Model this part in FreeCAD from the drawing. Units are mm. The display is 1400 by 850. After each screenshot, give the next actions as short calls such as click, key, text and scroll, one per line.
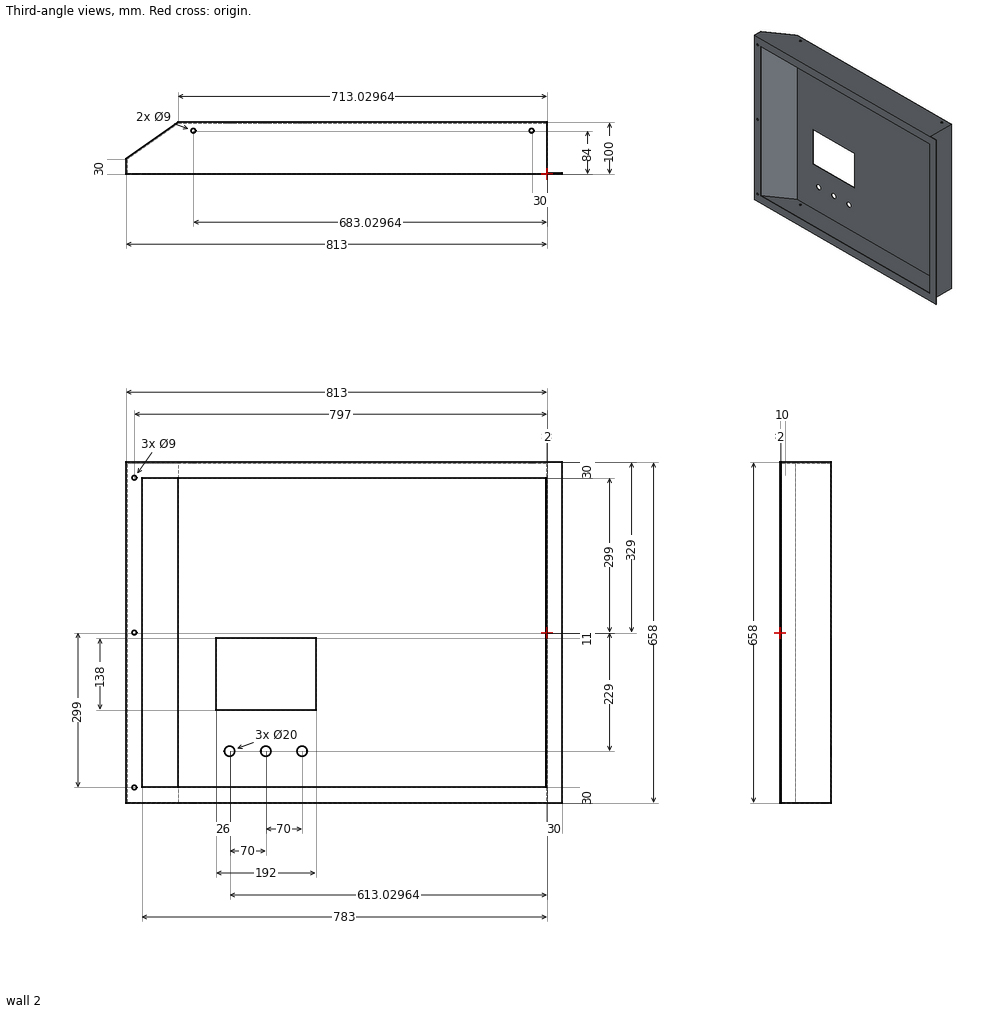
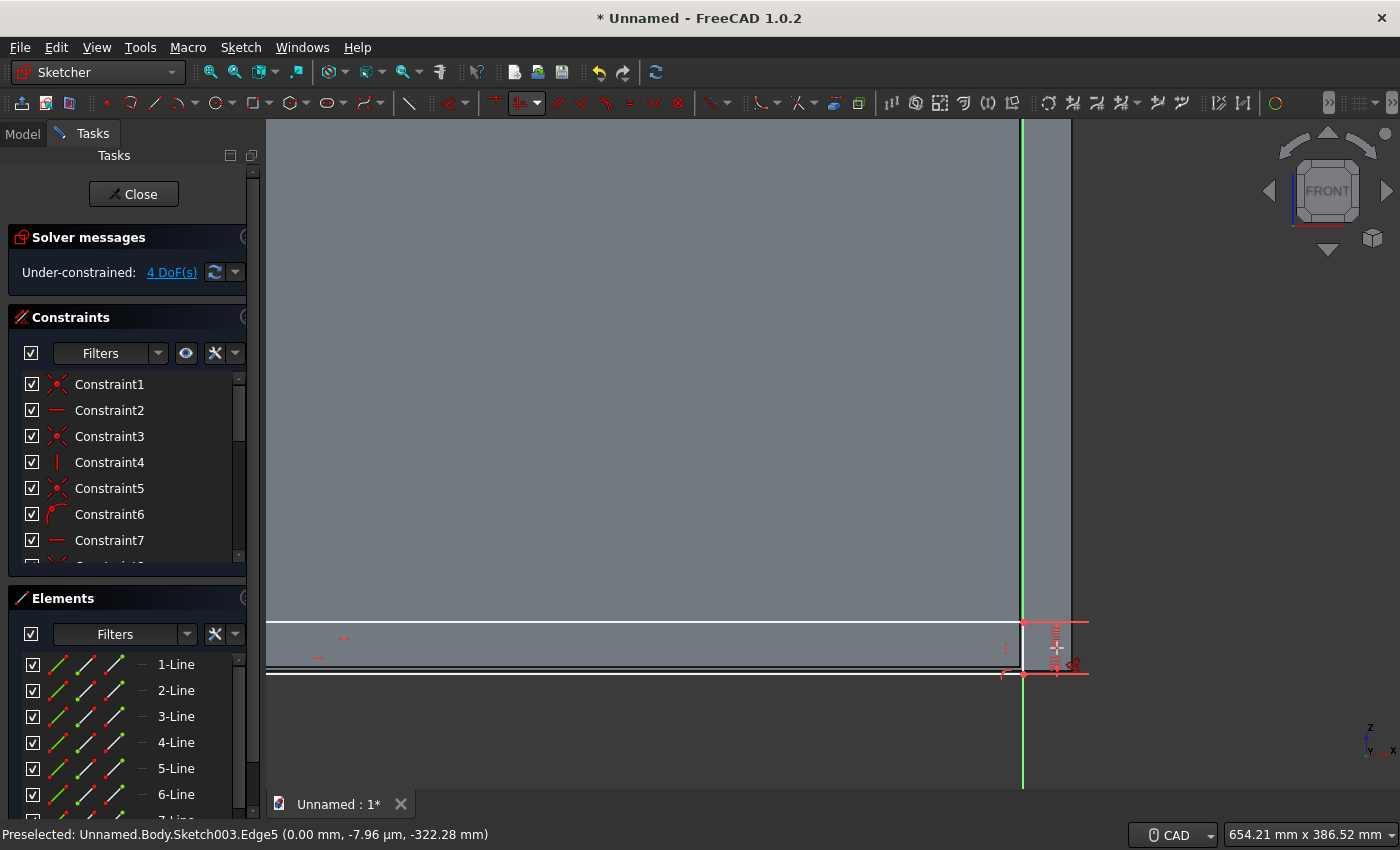
scroll(1024, 660, down, 5)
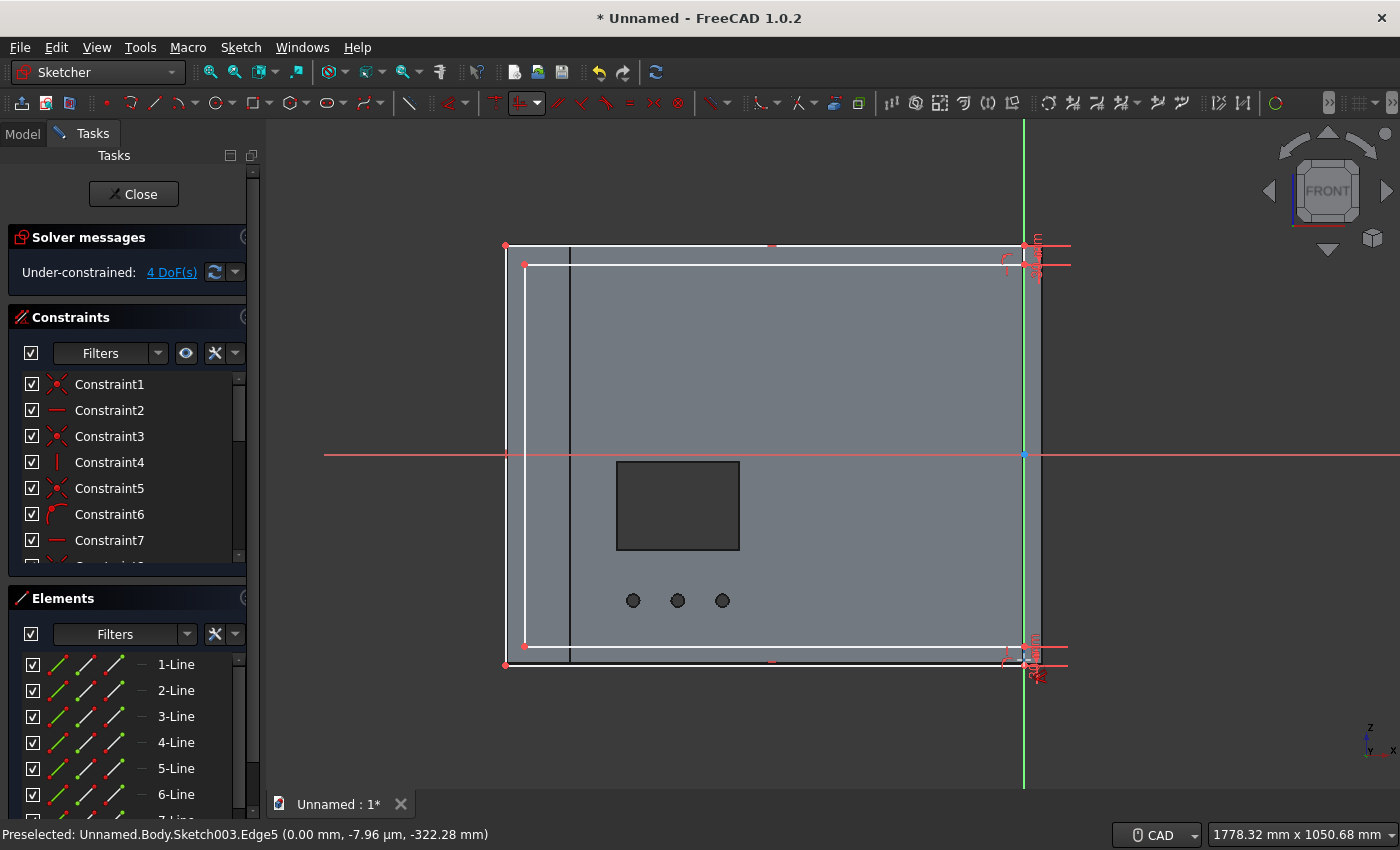
click(869, 246)
click(765, 212)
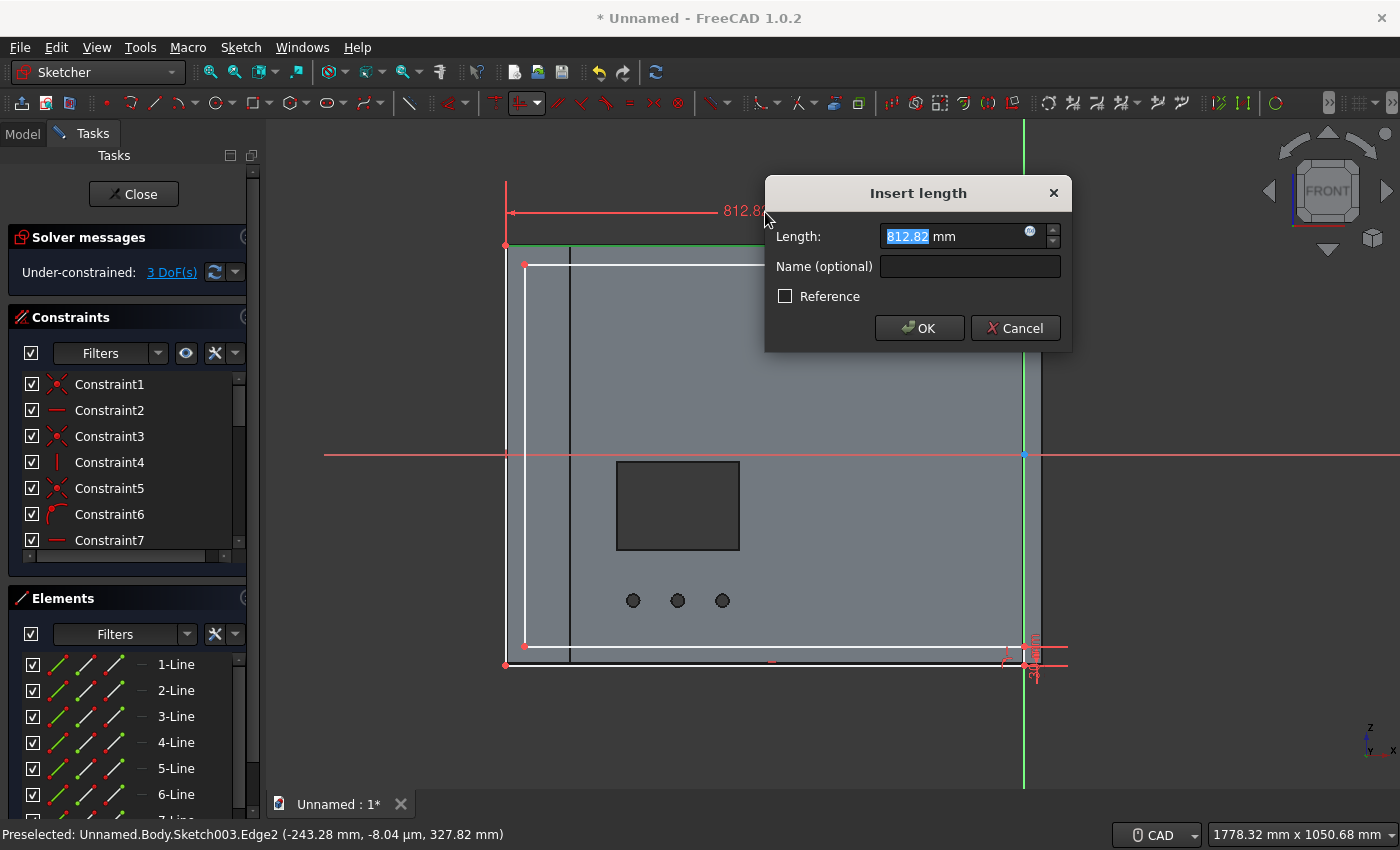
text(813)
key(Return)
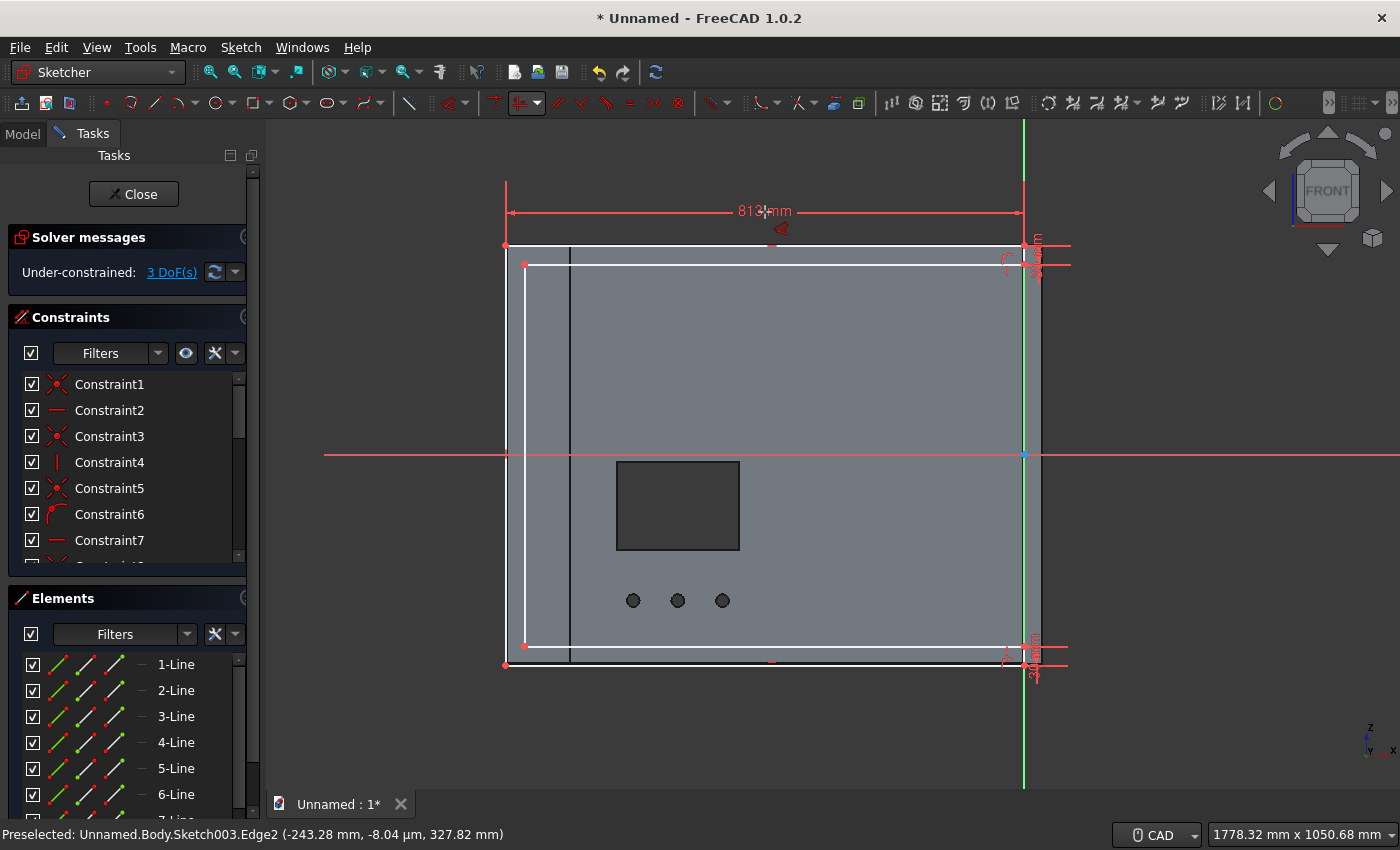
click(506, 372)
click(472, 359)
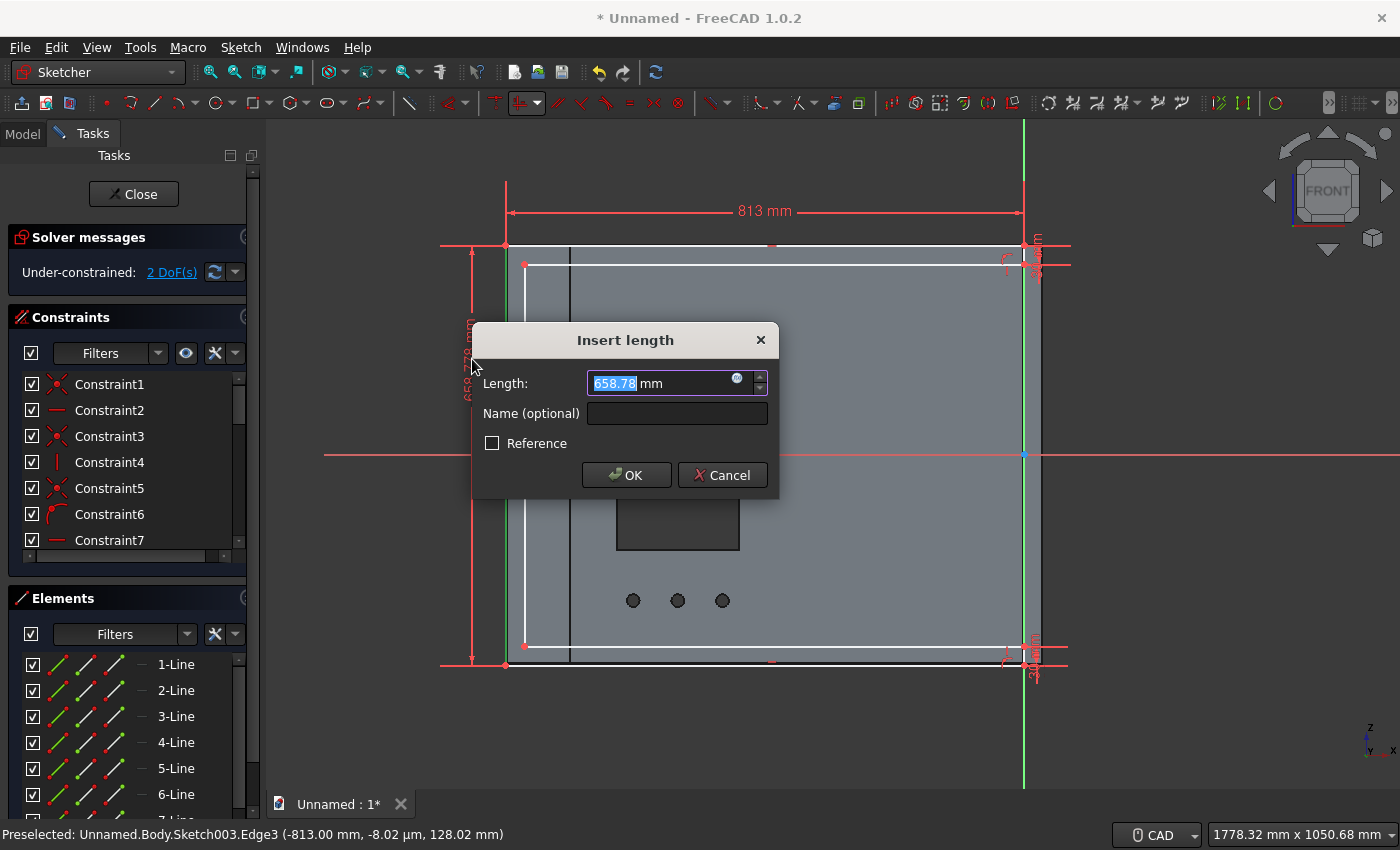
text(658)
key(Return)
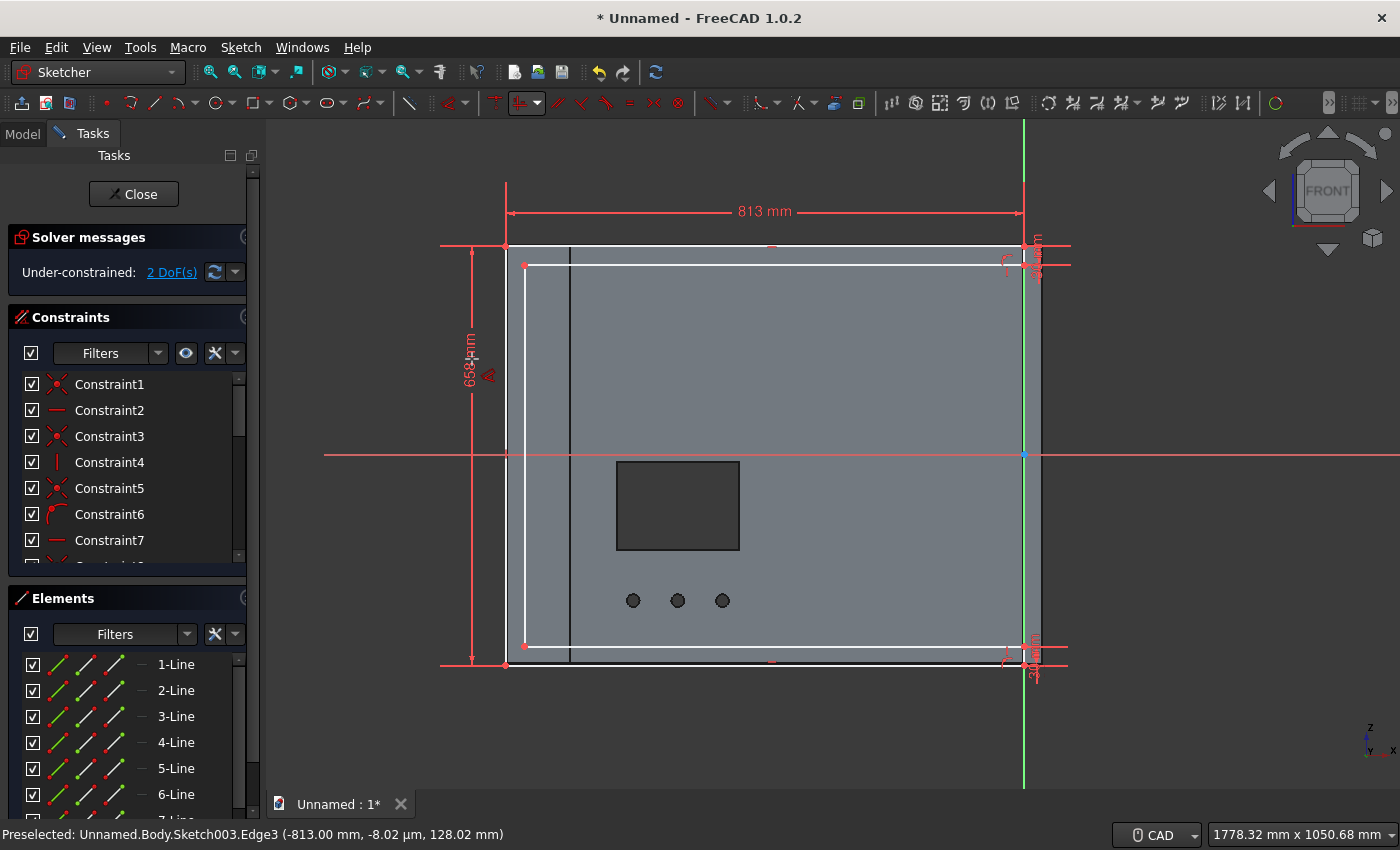
click(874, 647)
click(774, 681)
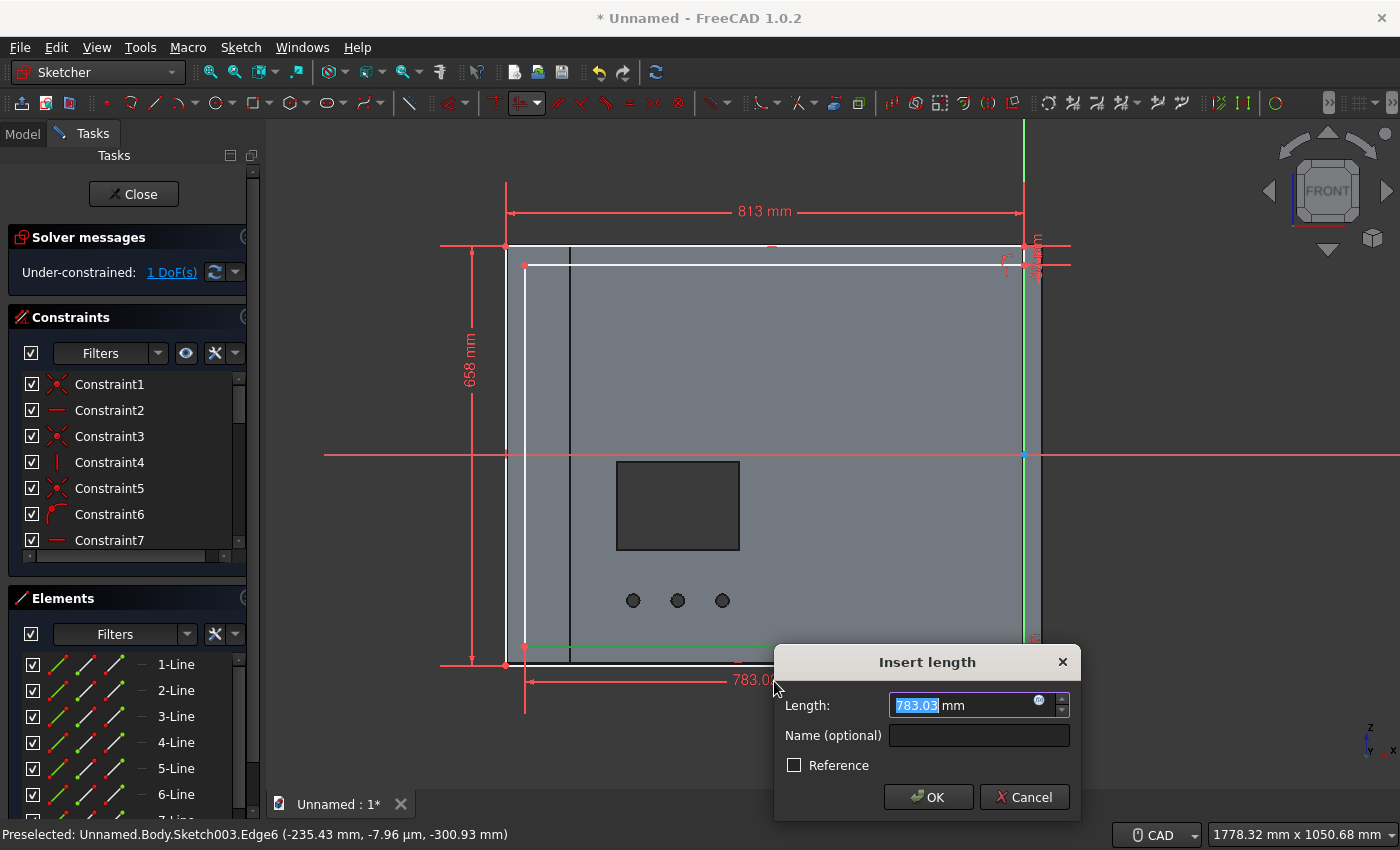
text(783)
key(Return)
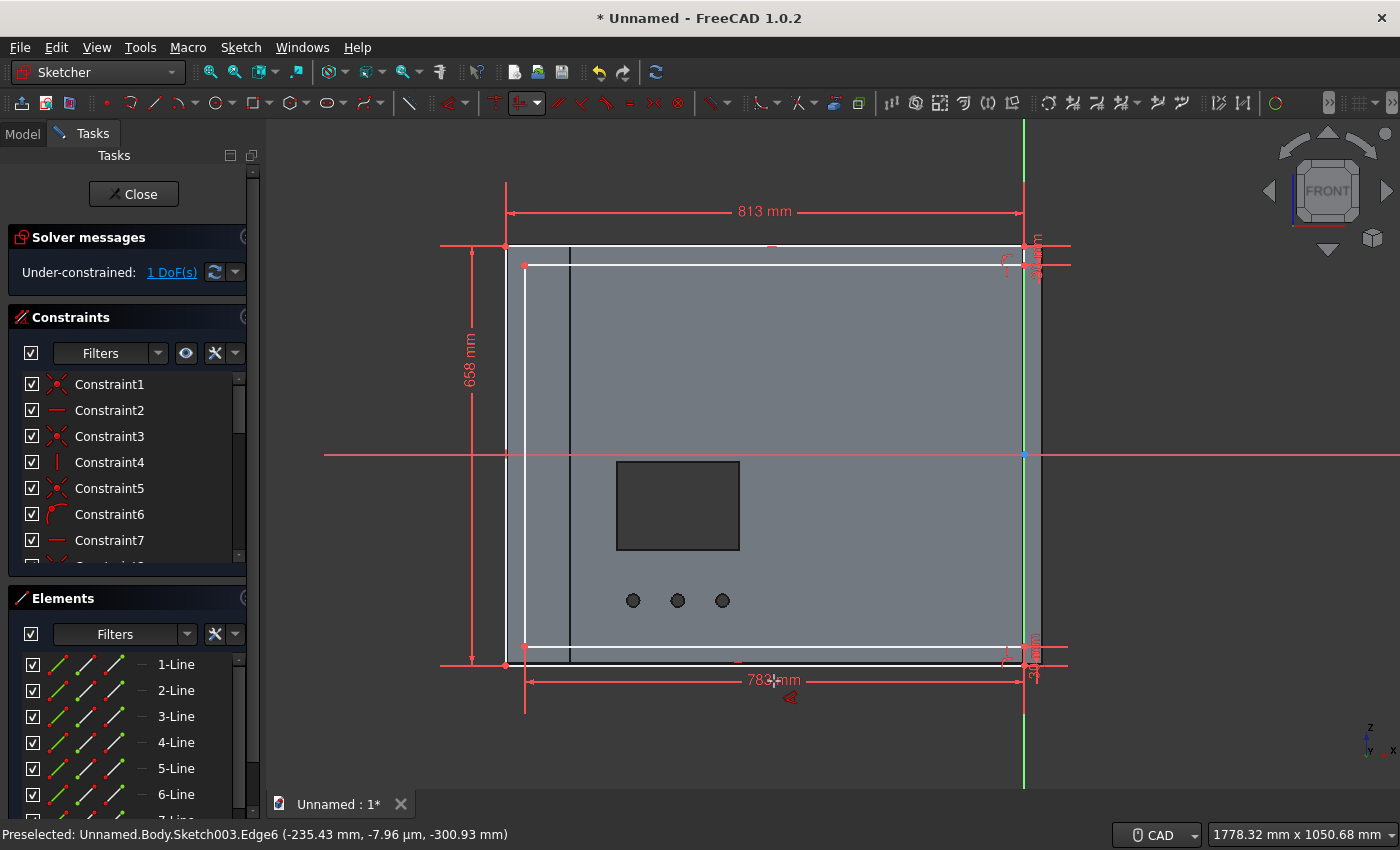
click(1024, 265)
click(1058, 360)